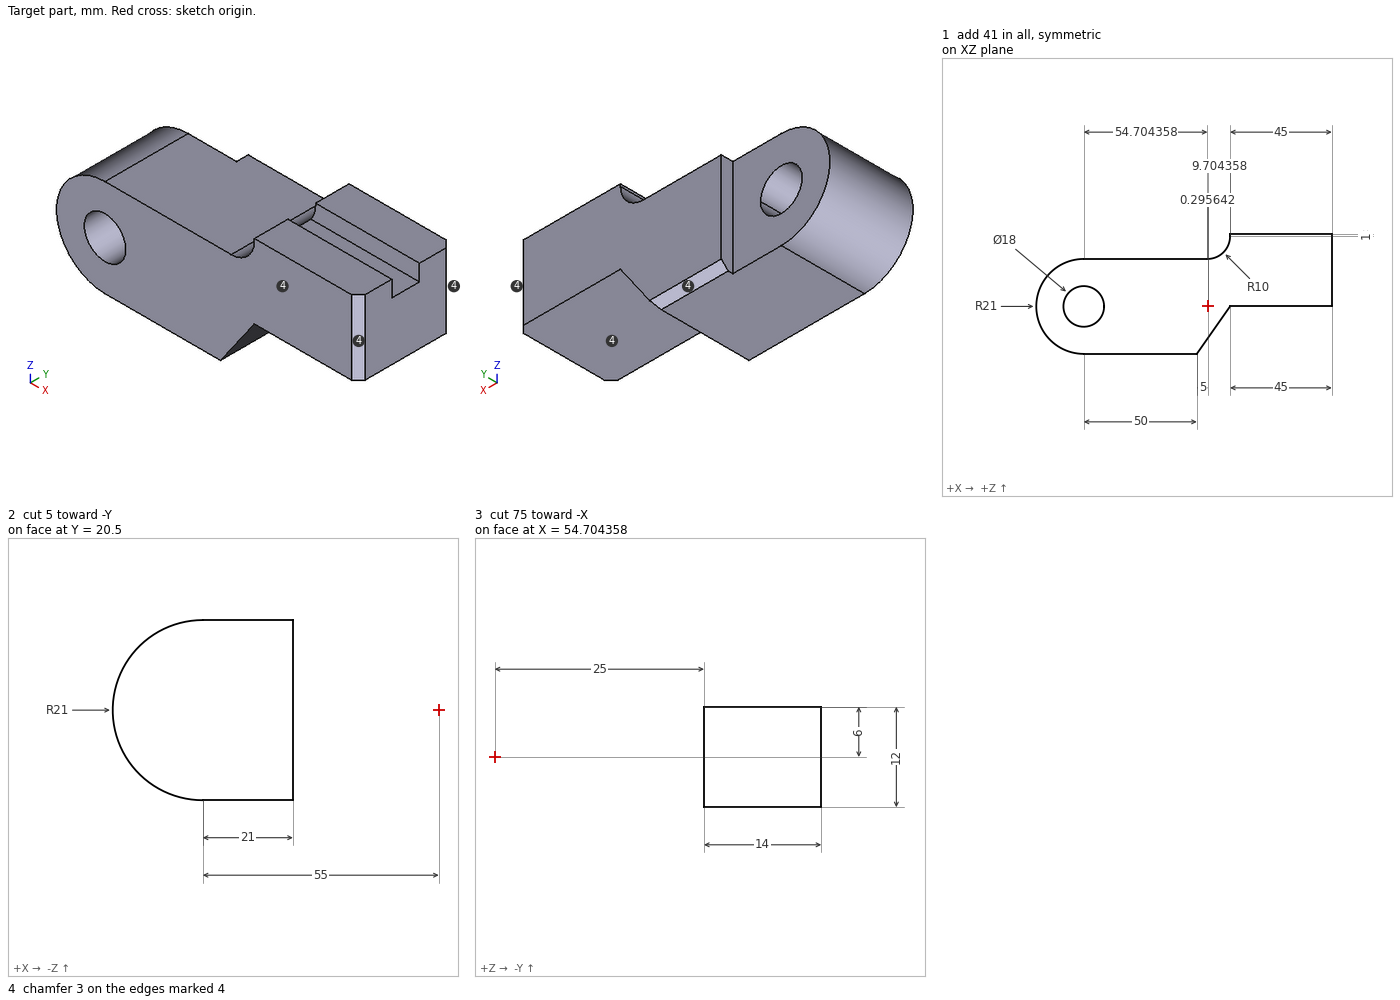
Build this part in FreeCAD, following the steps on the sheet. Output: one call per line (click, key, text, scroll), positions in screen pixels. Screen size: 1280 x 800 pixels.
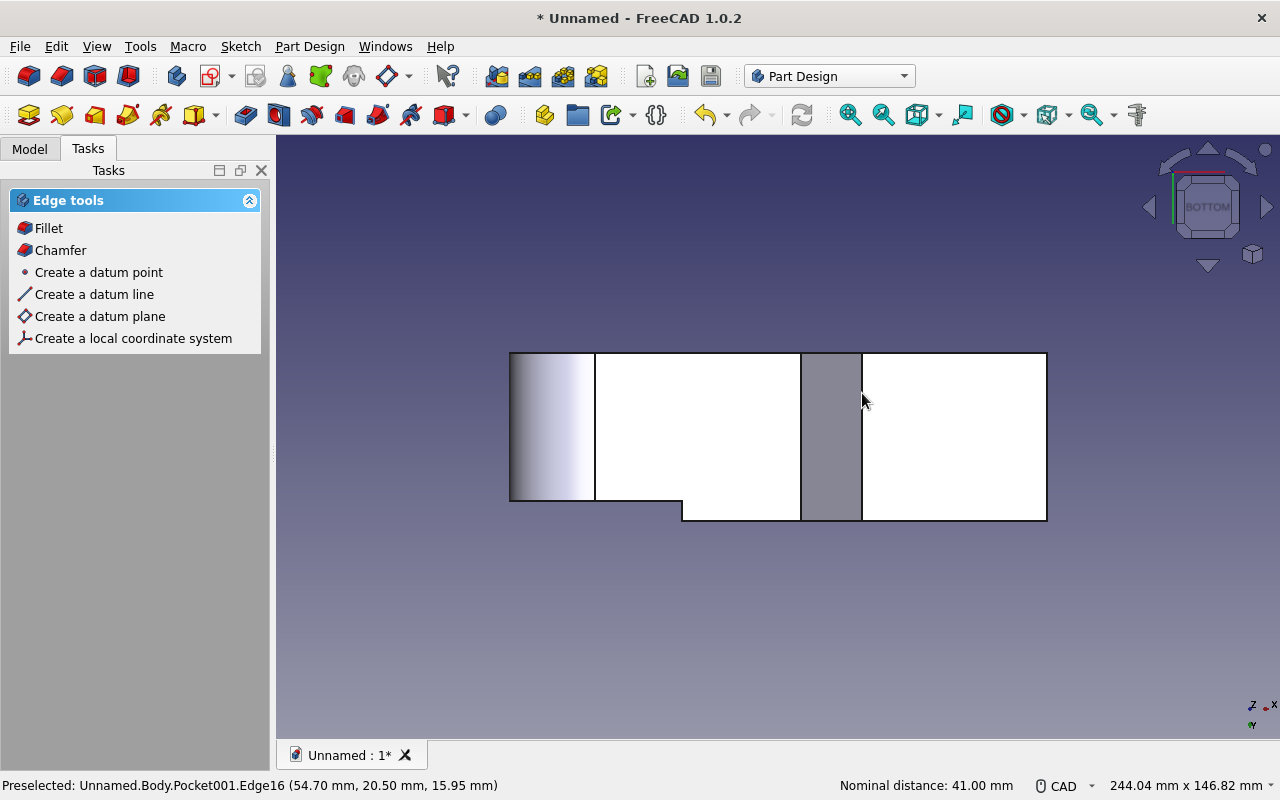
key(4)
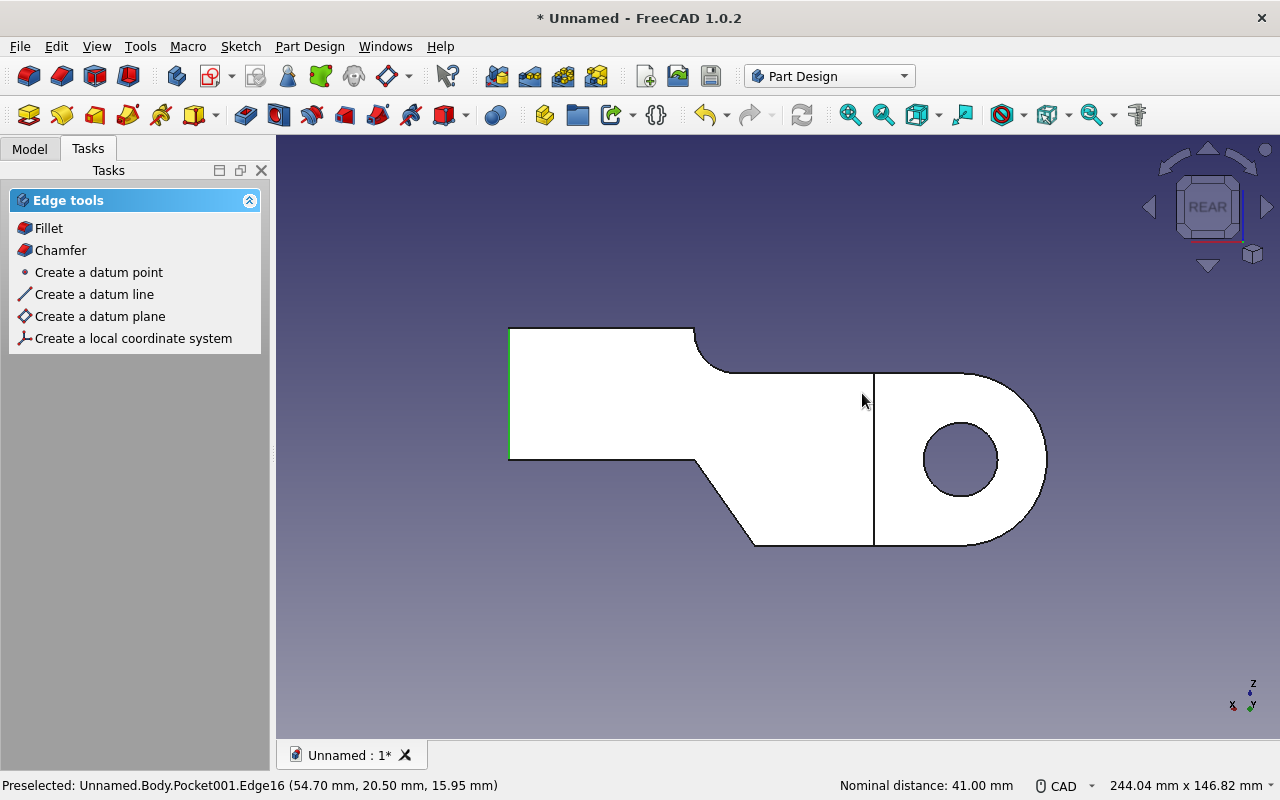
click(815, 545, ctrl)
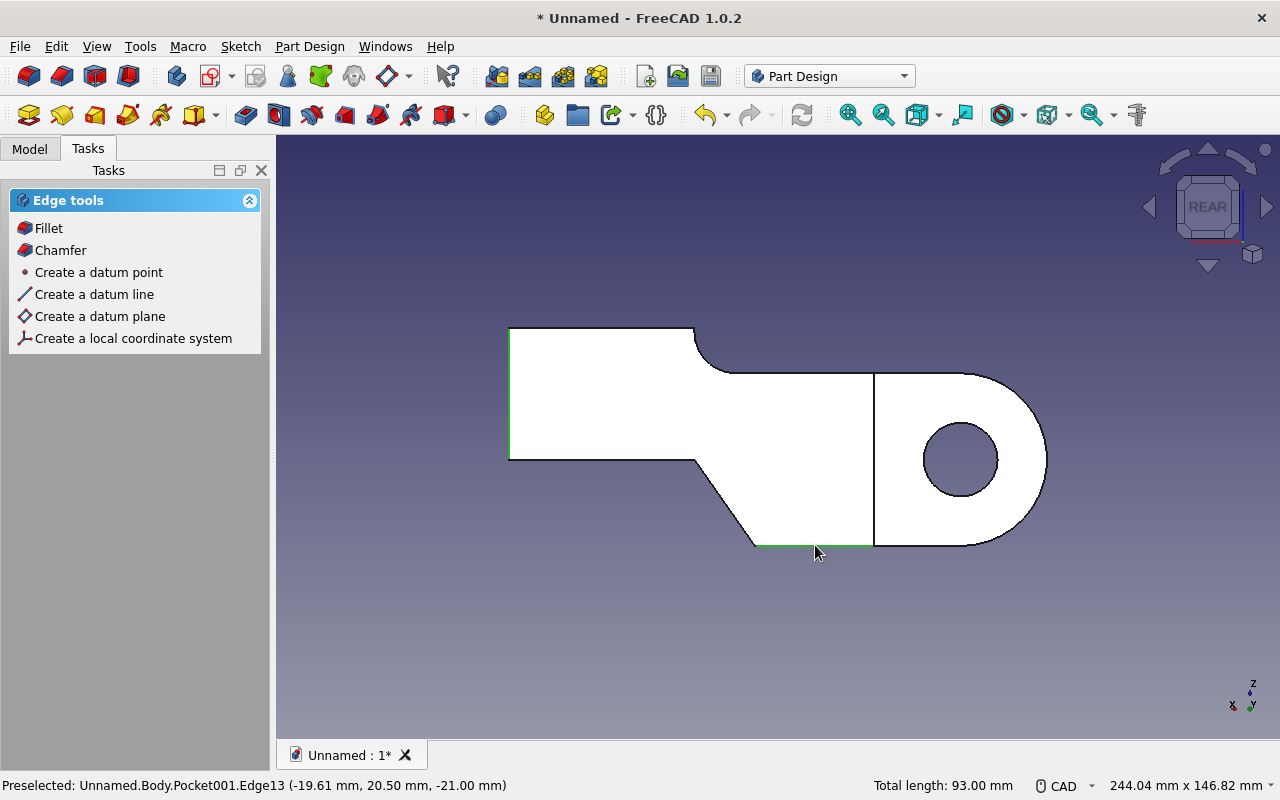
click(62, 76)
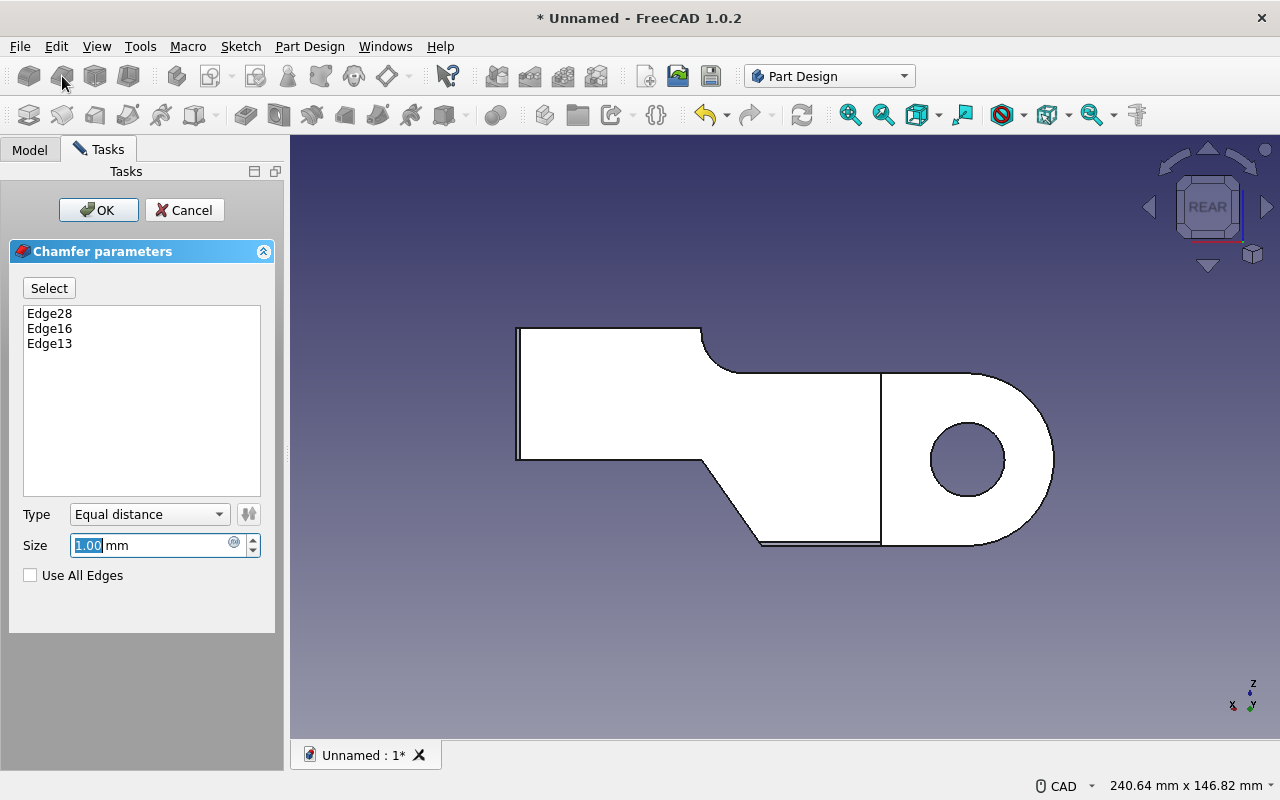
text(3)
key(Tab)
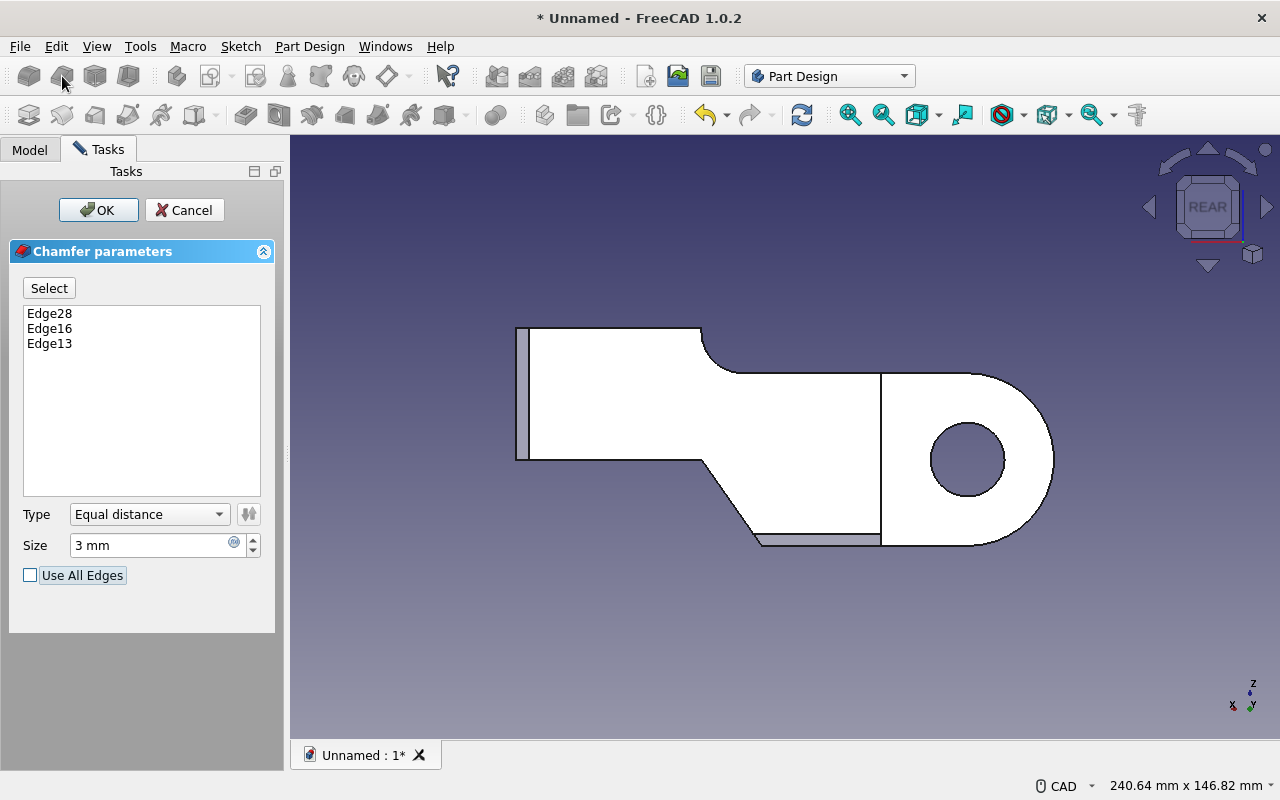
click(99, 210)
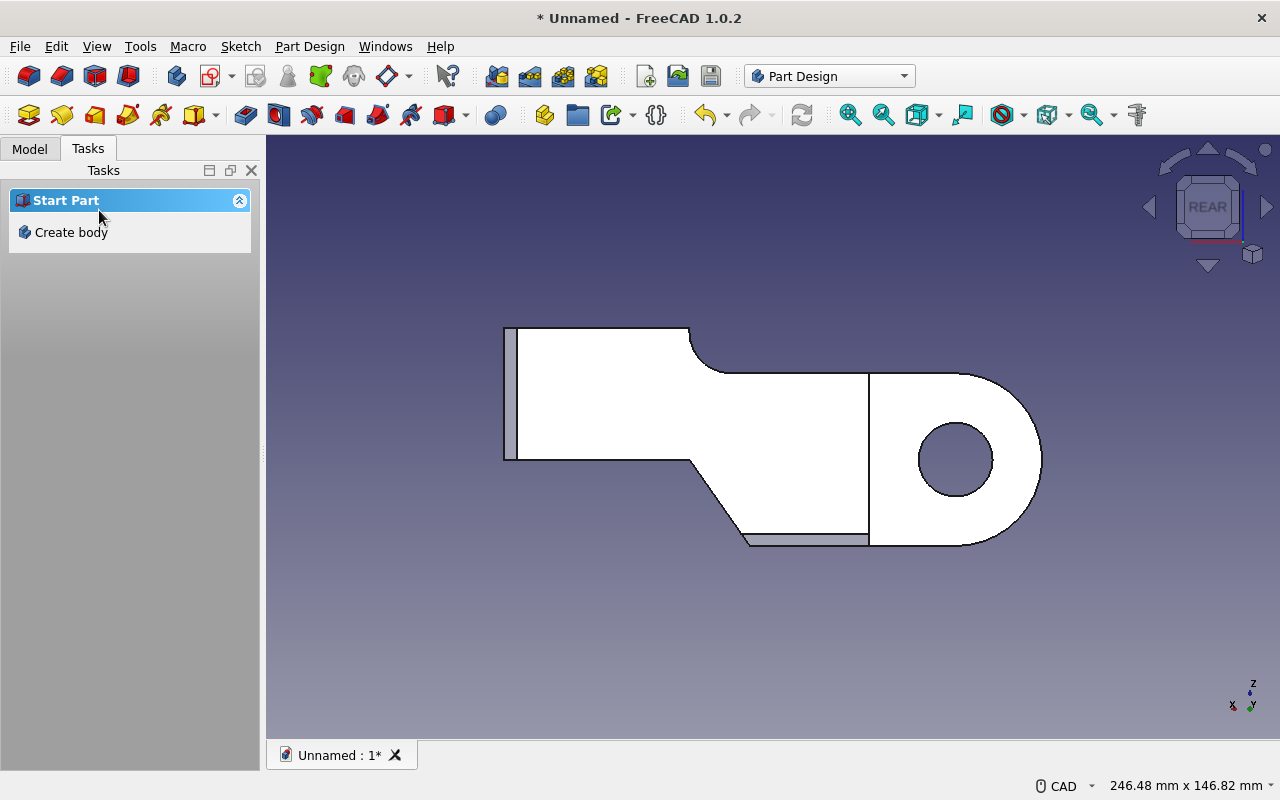
key(0)